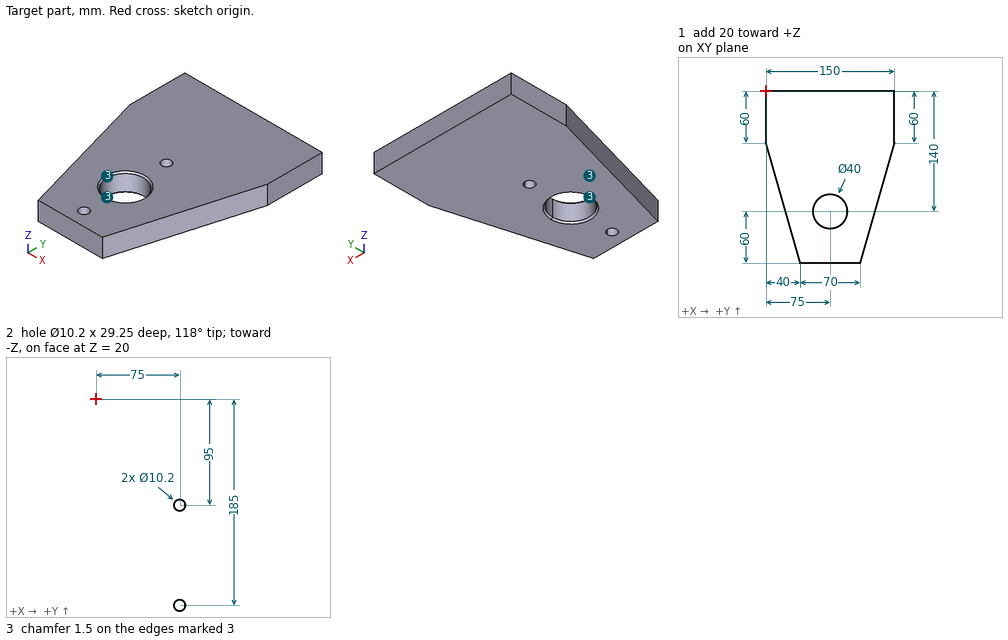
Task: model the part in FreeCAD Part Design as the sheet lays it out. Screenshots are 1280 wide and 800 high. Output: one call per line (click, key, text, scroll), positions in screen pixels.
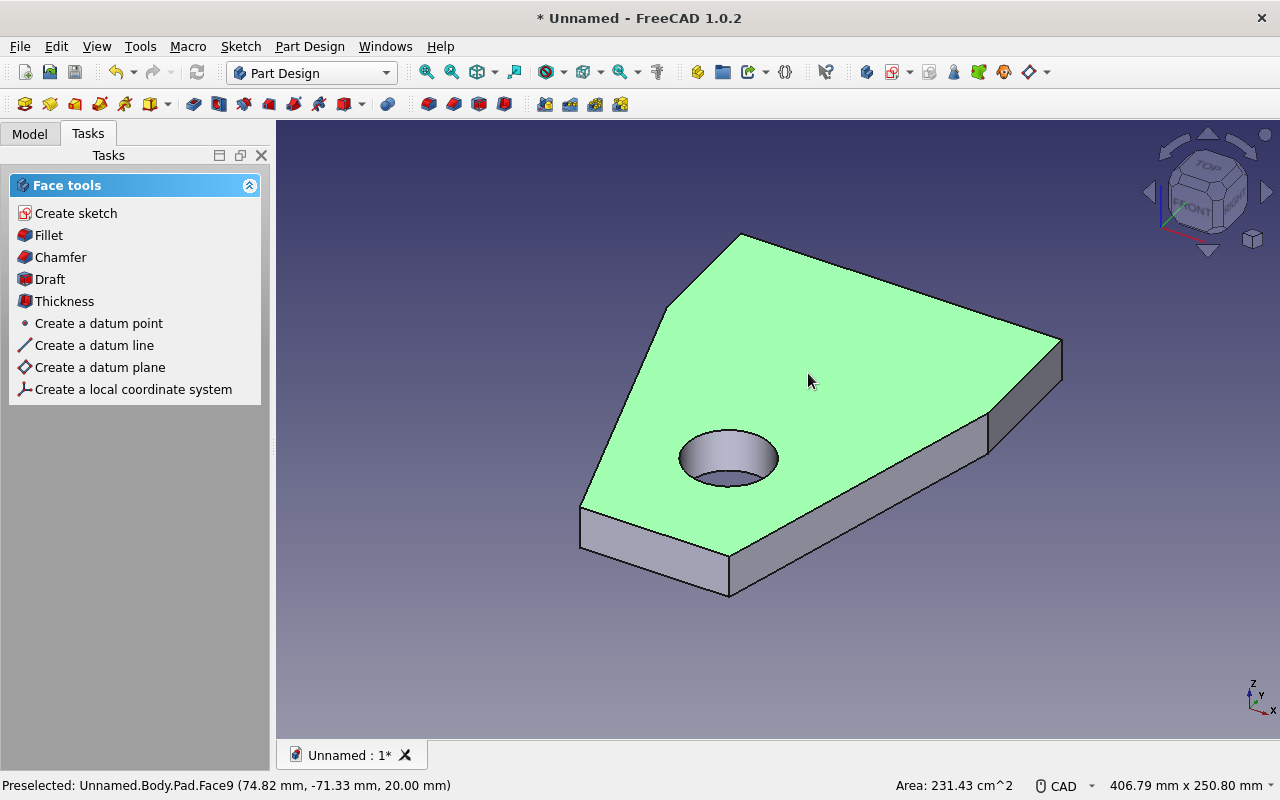
click(892, 72)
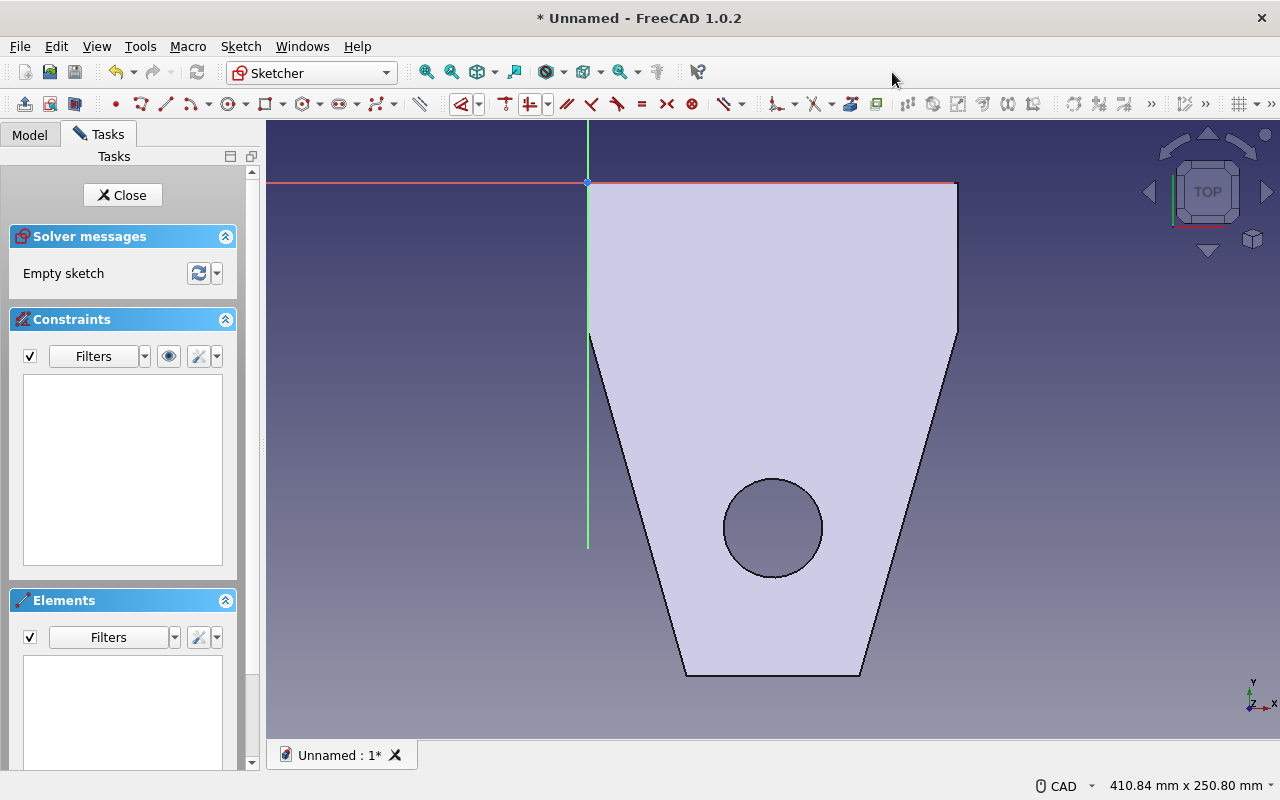
click(228, 104)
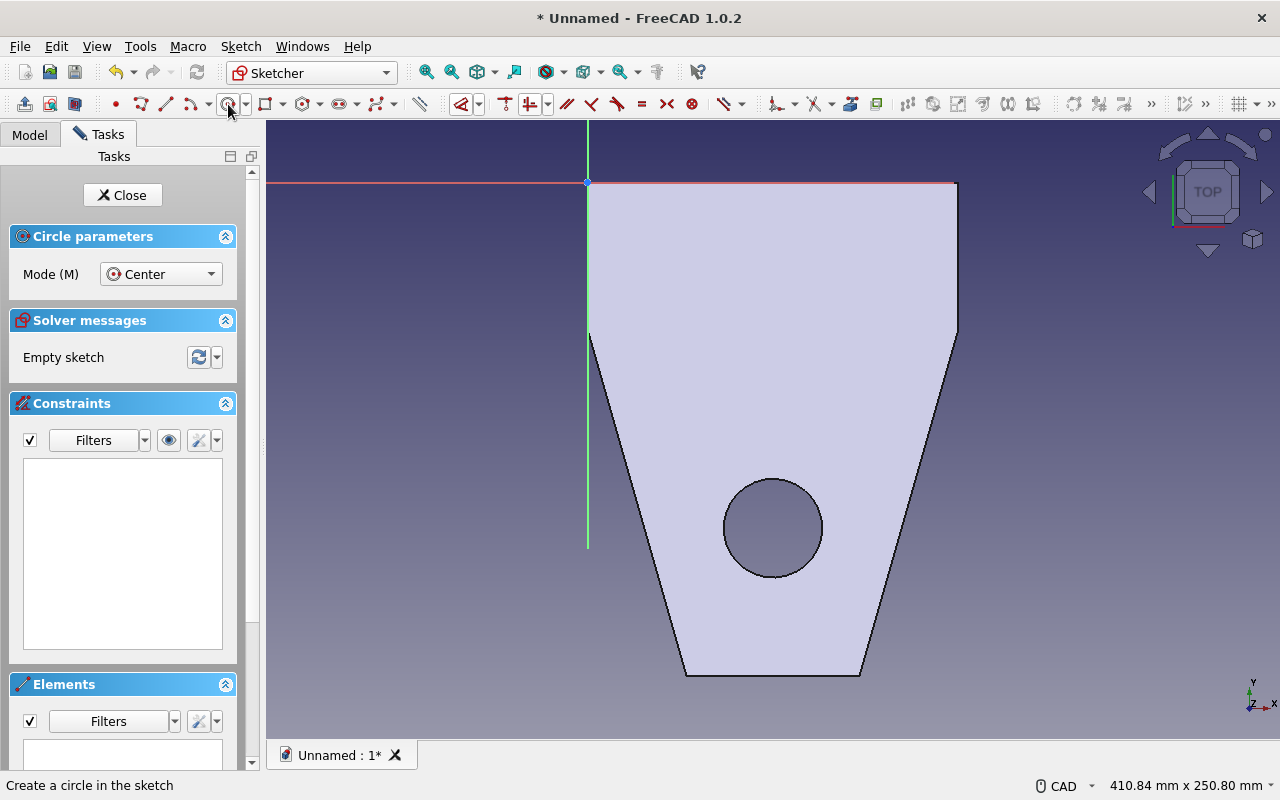
scroll(773, 417, up, 3)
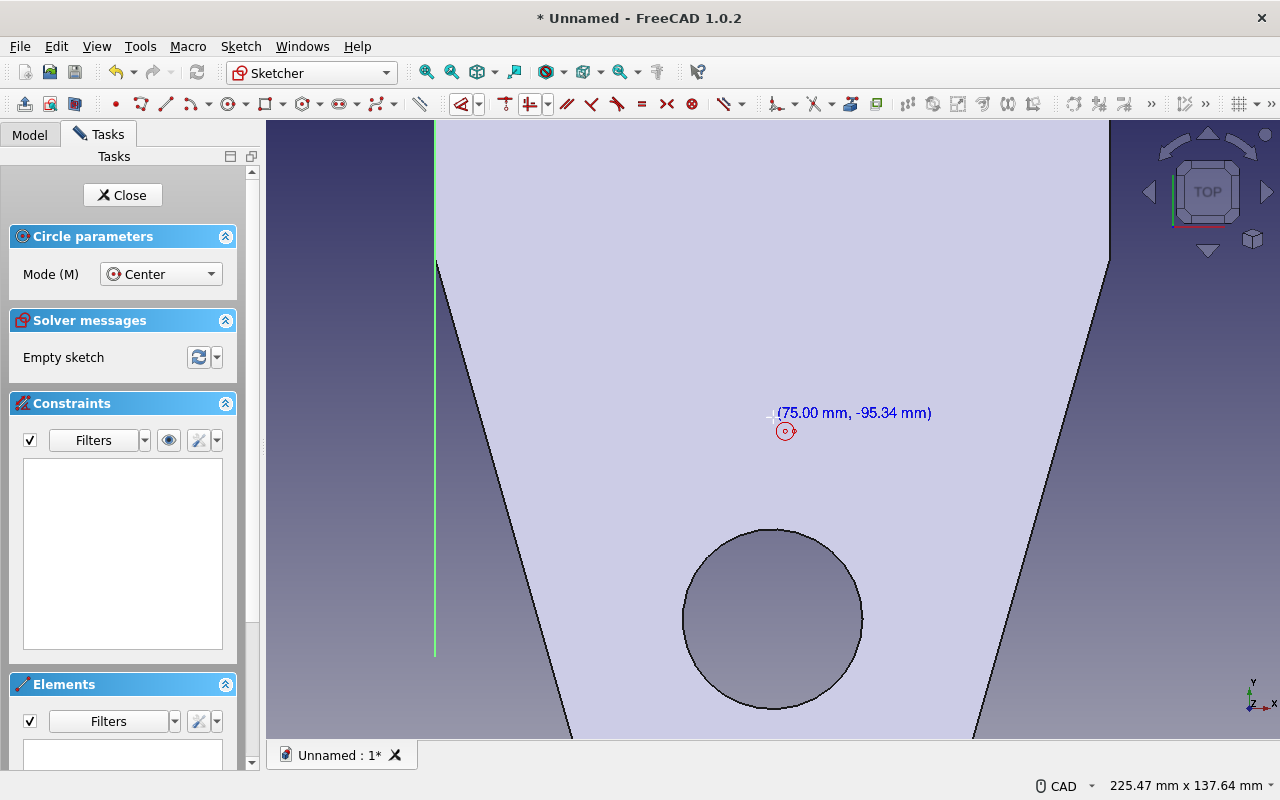
click(773, 417)
click(789, 401)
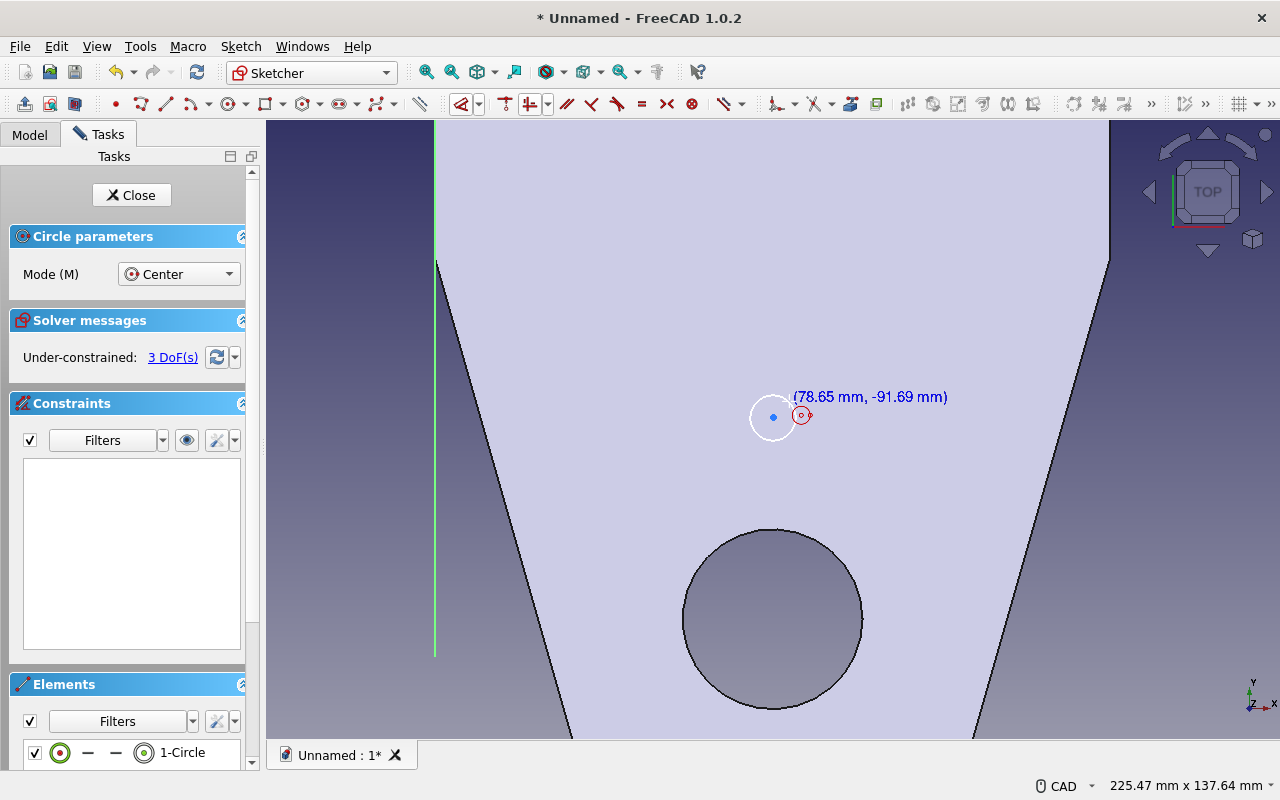
scroll(777, 440, down, 4)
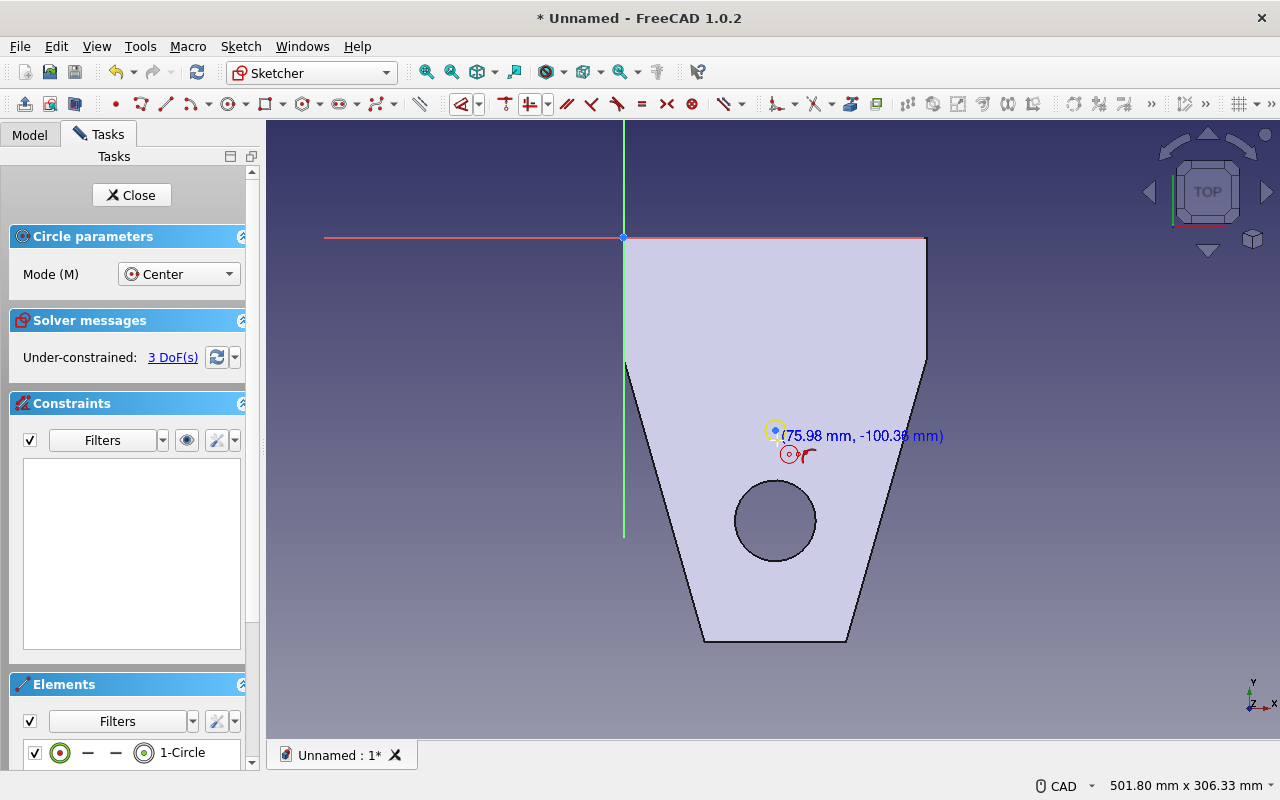
scroll(775, 612, up, 4)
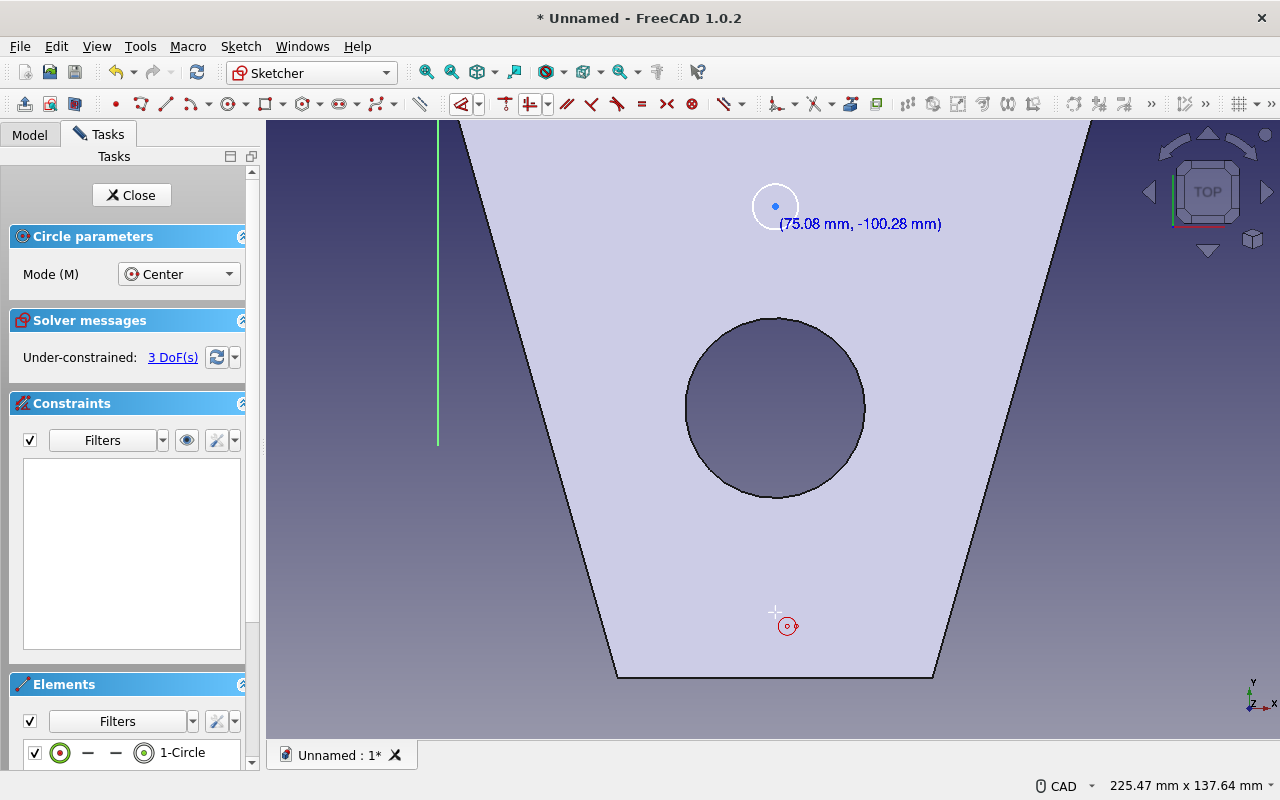
click(775, 611)
click(791, 594)
key(Escape)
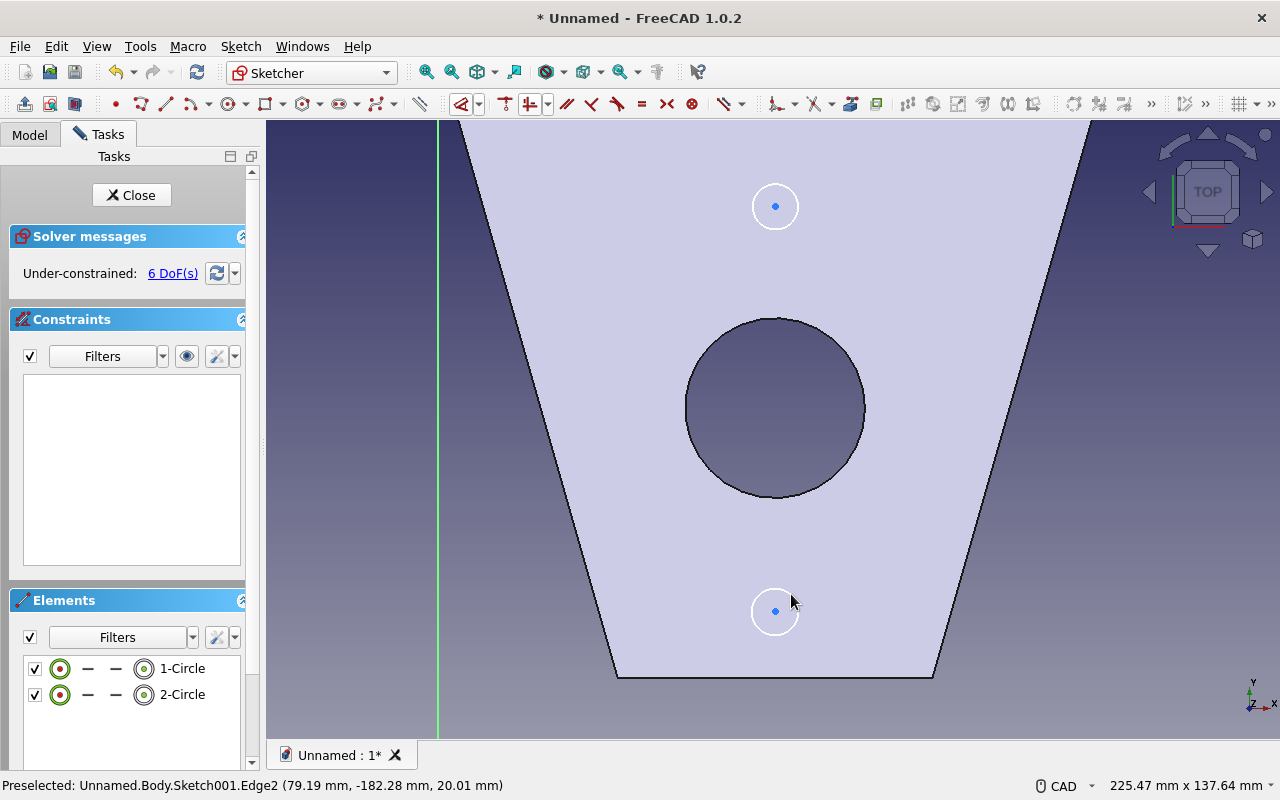
click(791, 191)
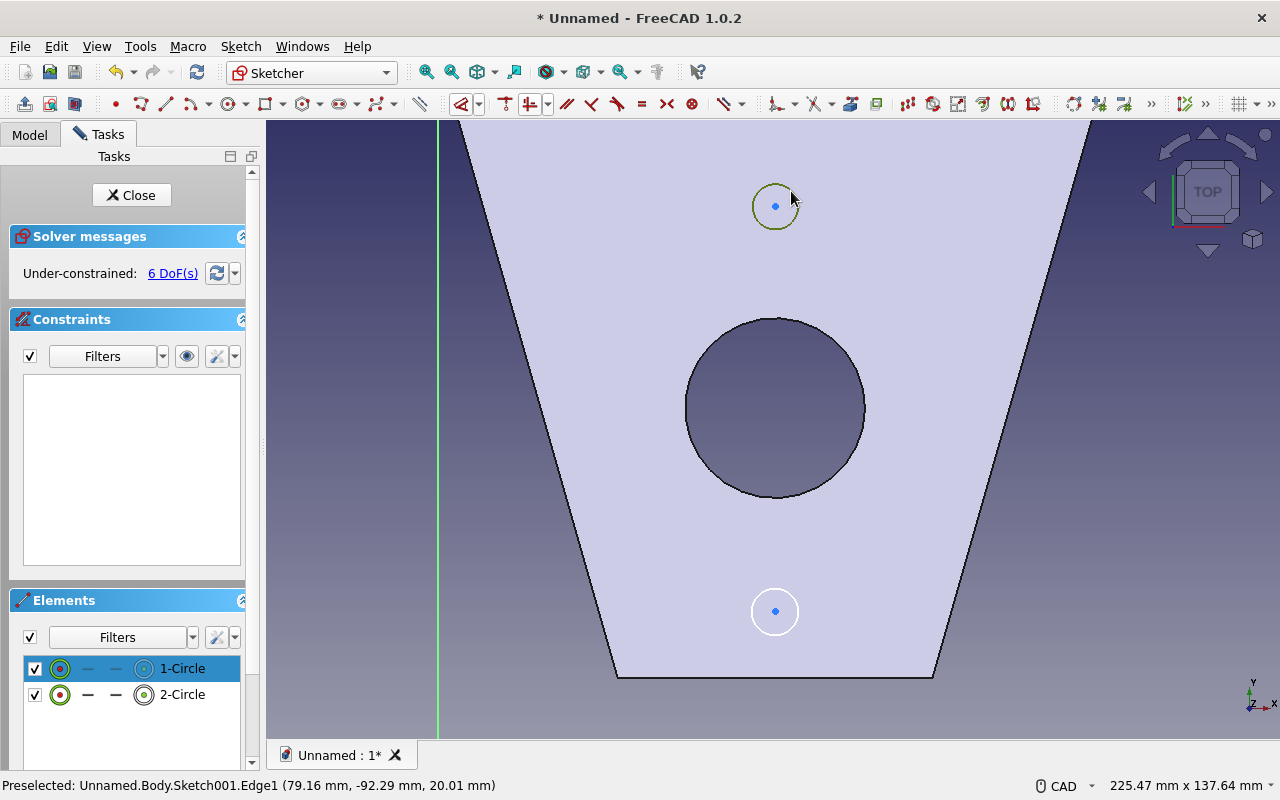
click(791, 595)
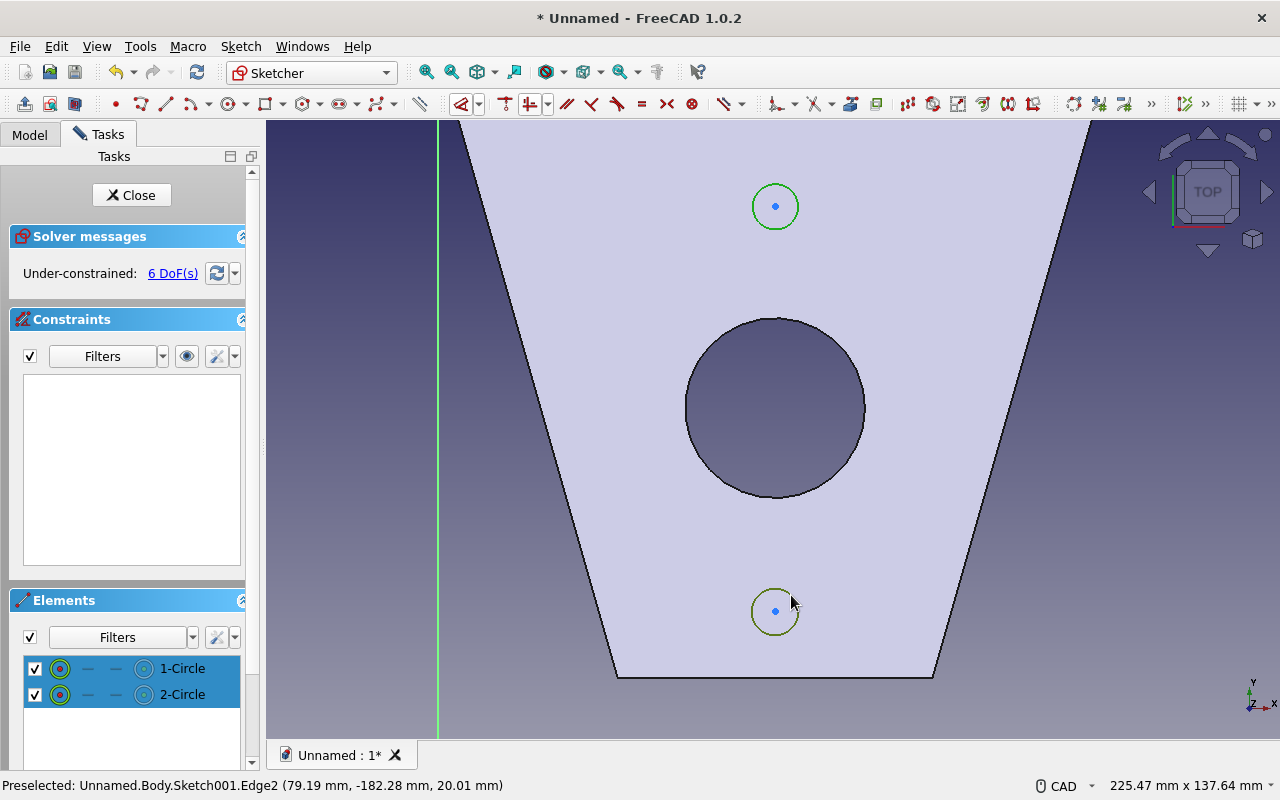
click(642, 104)